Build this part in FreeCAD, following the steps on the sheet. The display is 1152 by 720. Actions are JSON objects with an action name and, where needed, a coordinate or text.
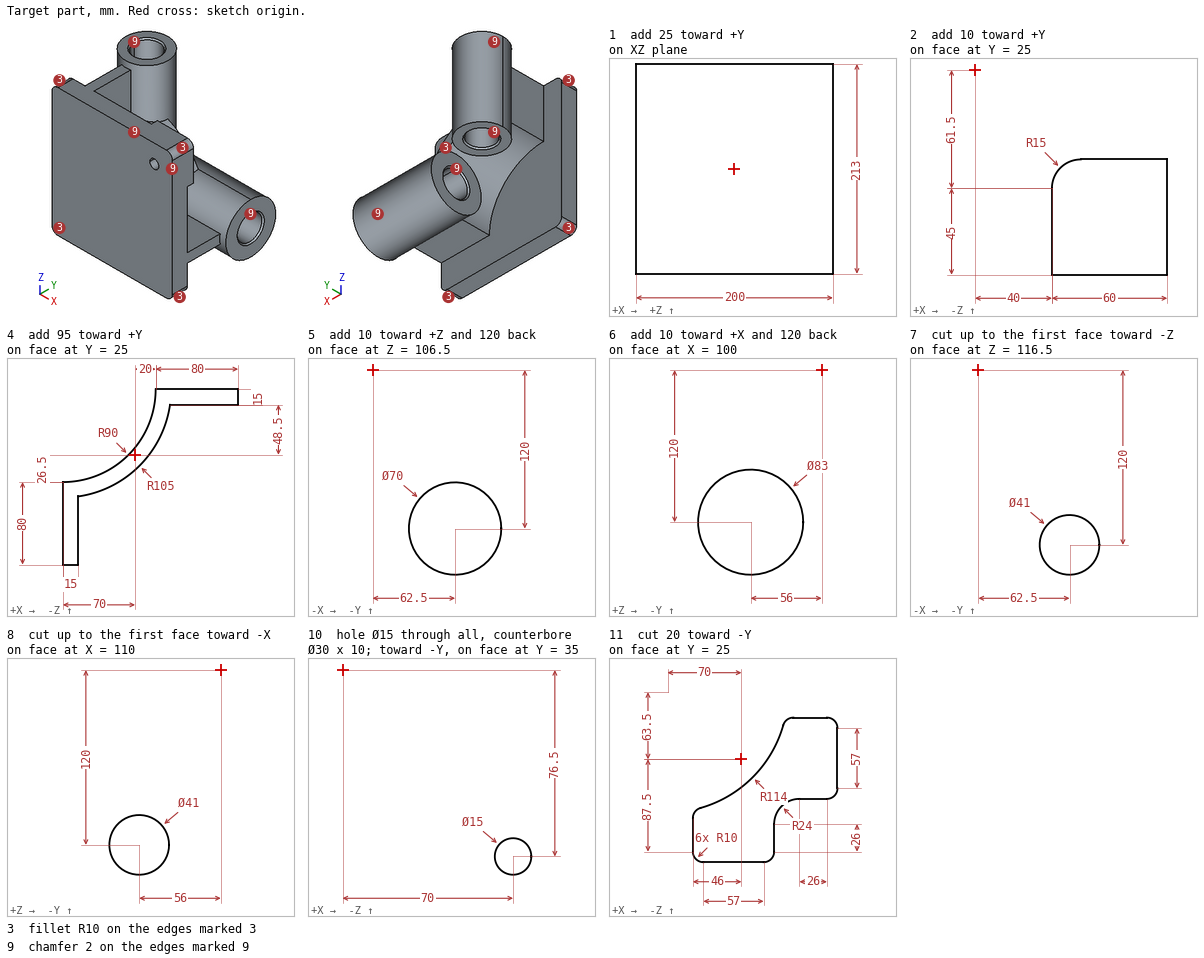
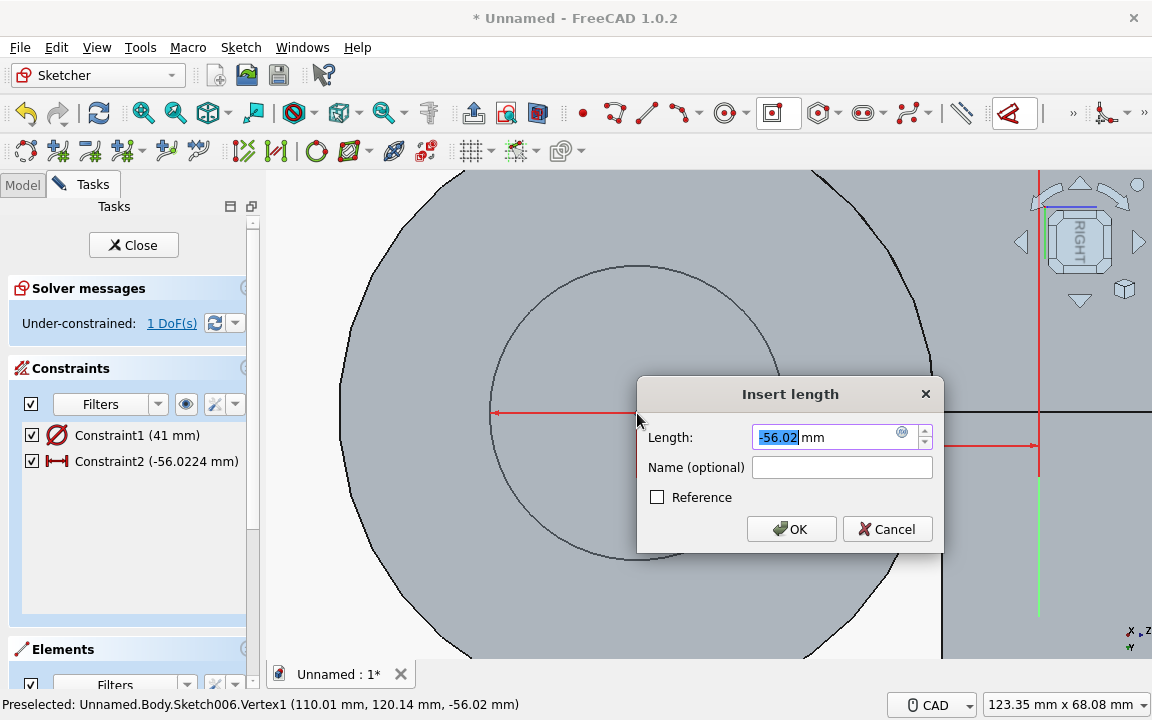
{"action": "type", "text": "-56"}
{"action": "key", "text": "Return"}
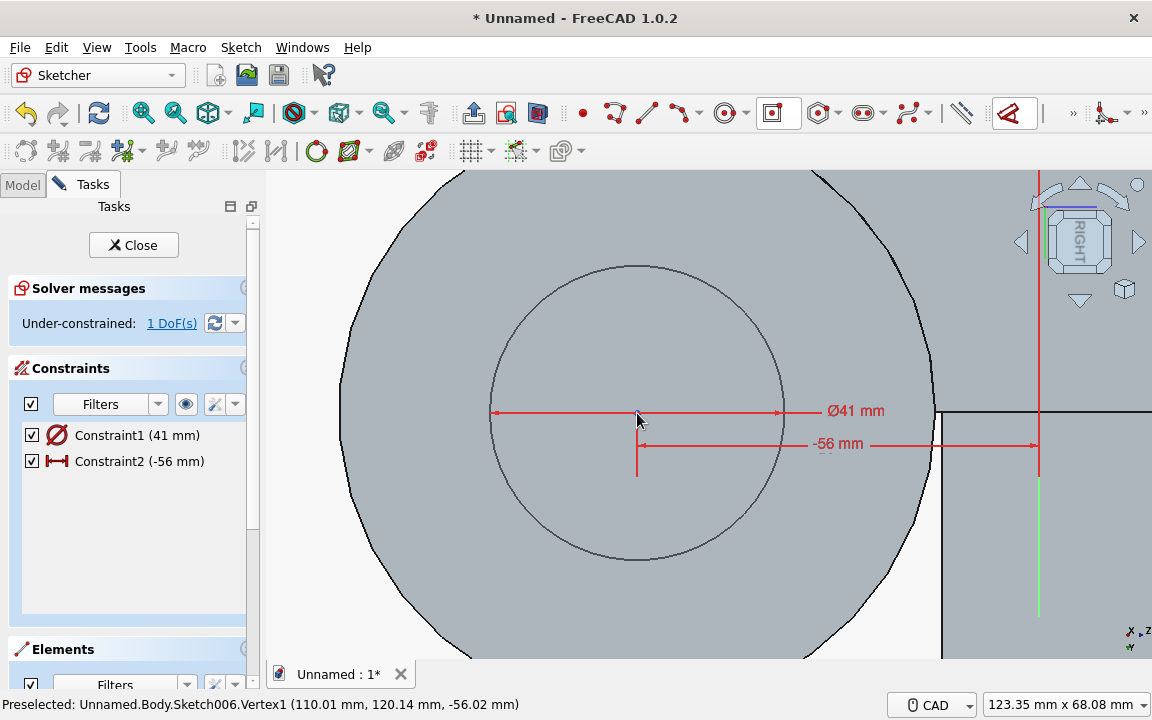
{"action": "left_click", "coordinate": [637, 413]}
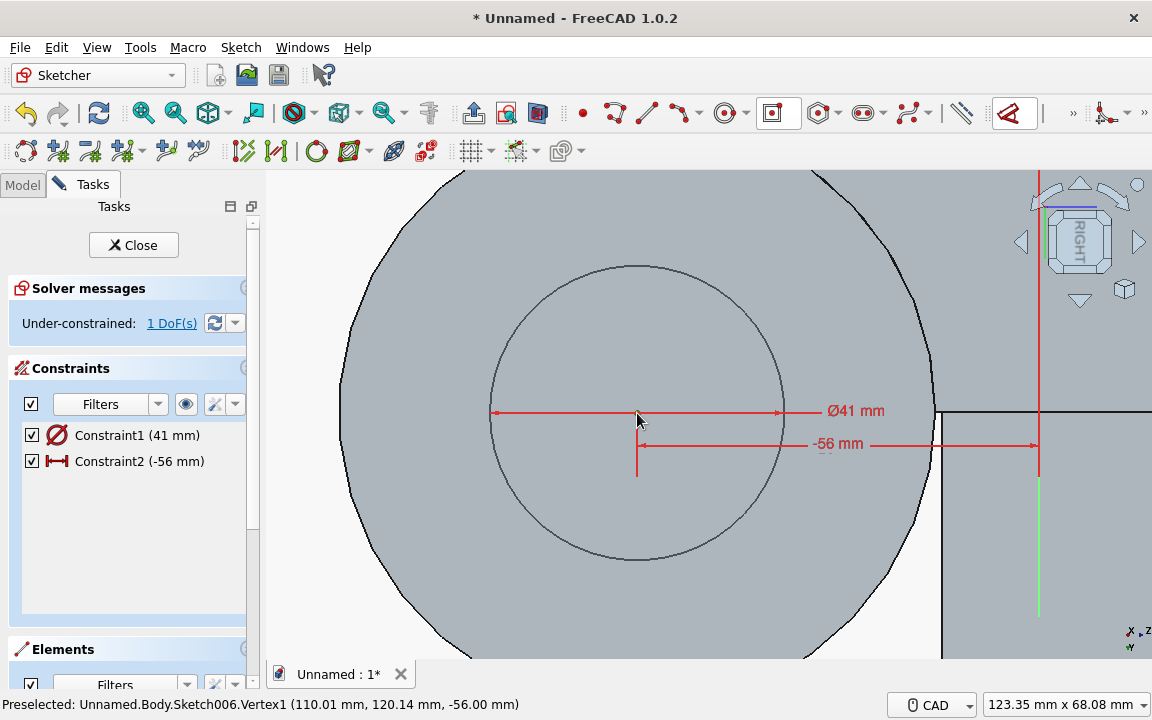
{"action": "left_click", "coordinate": [1032, 114]}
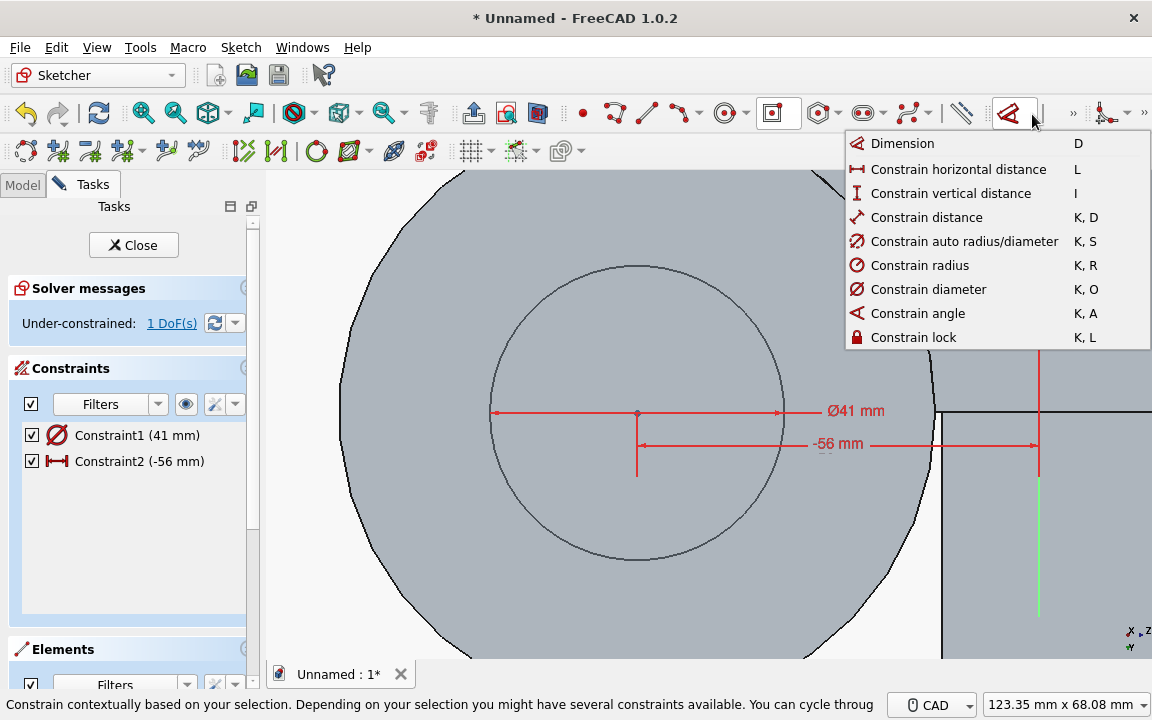
{"action": "left_click", "coordinate": [998, 193]}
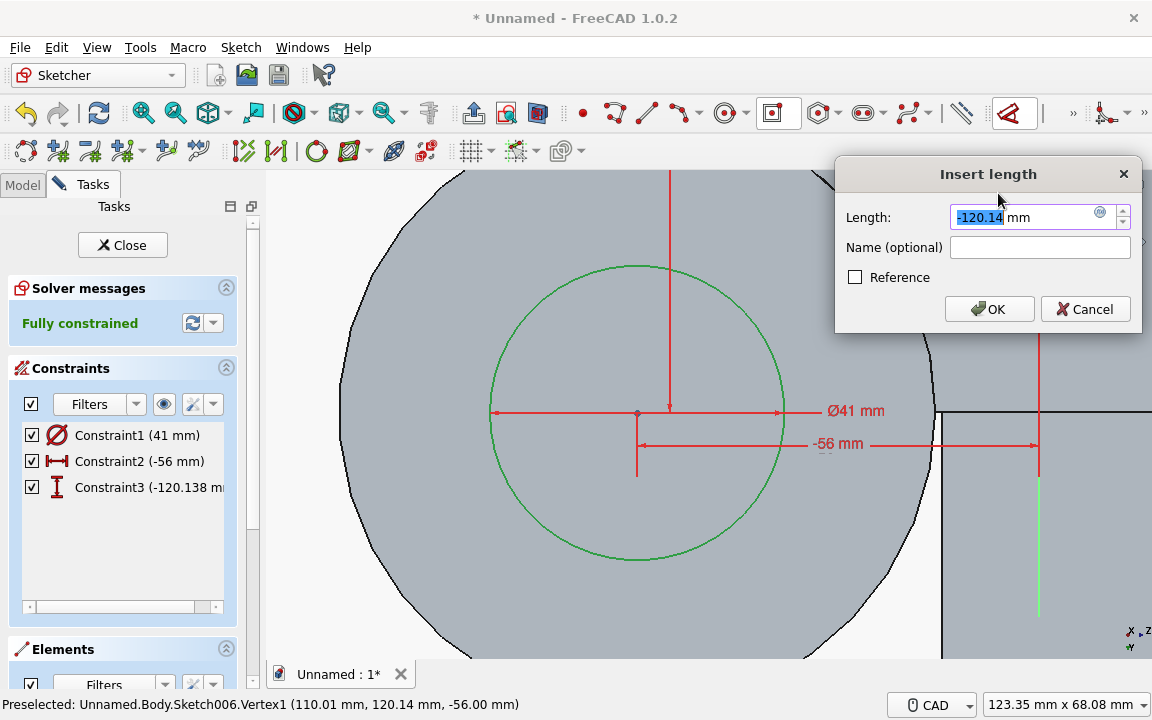
{"action": "type", "text": "-120"}
{"action": "key", "text": "Return"}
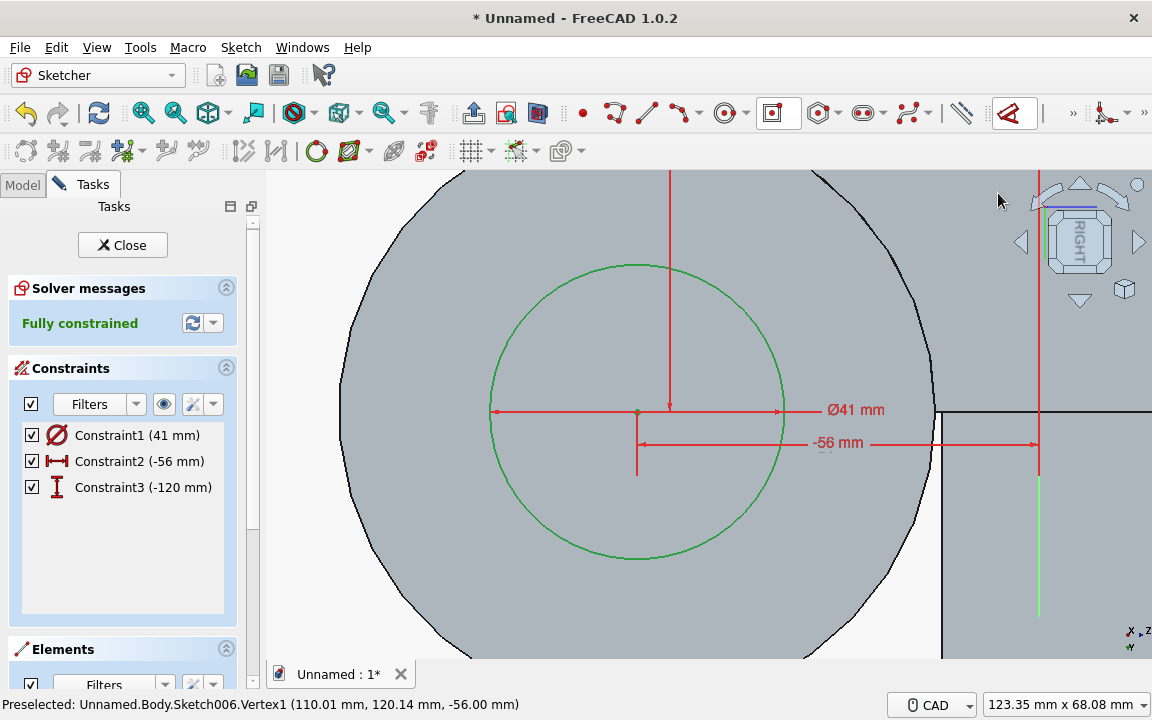
{"action": "left_click", "coordinate": [123, 245]}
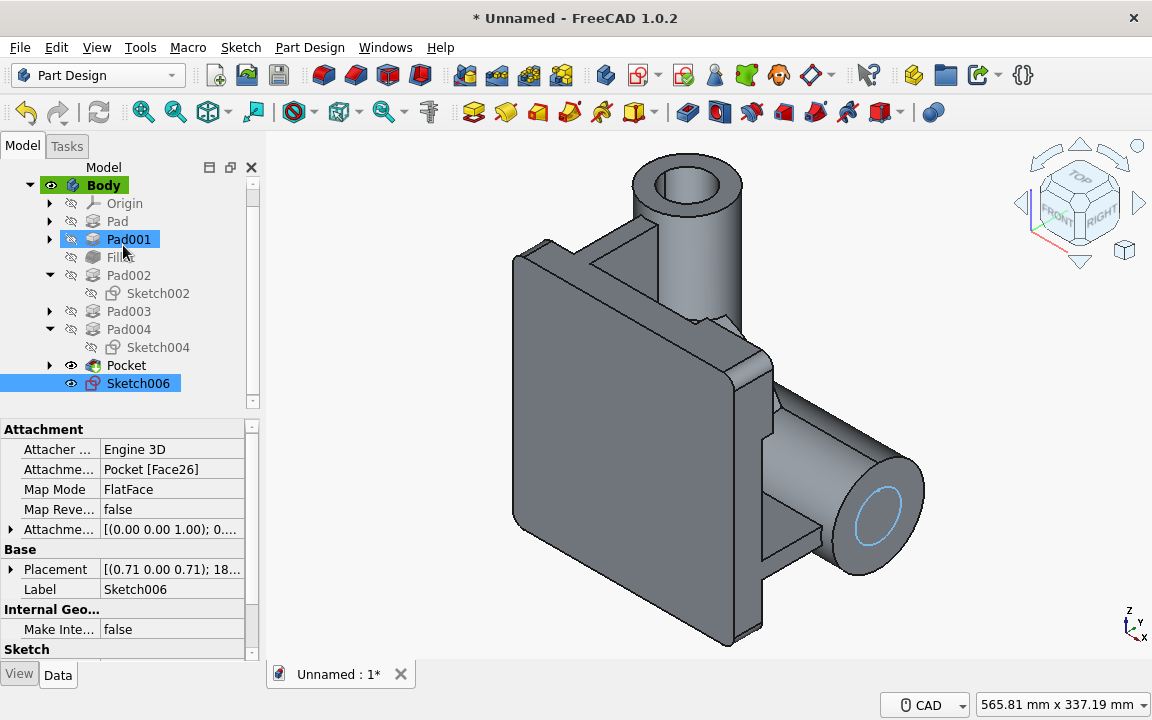
{"action": "left_click", "coordinate": [688, 112]}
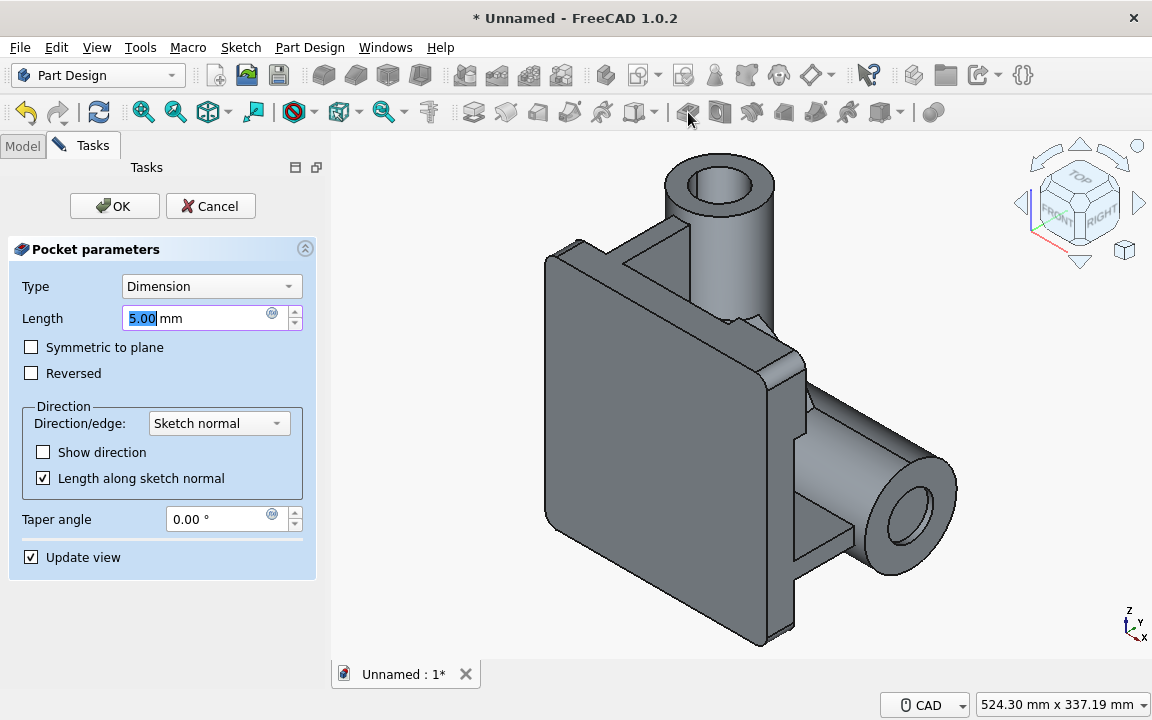
{"action": "left_click", "coordinate": [212, 286]}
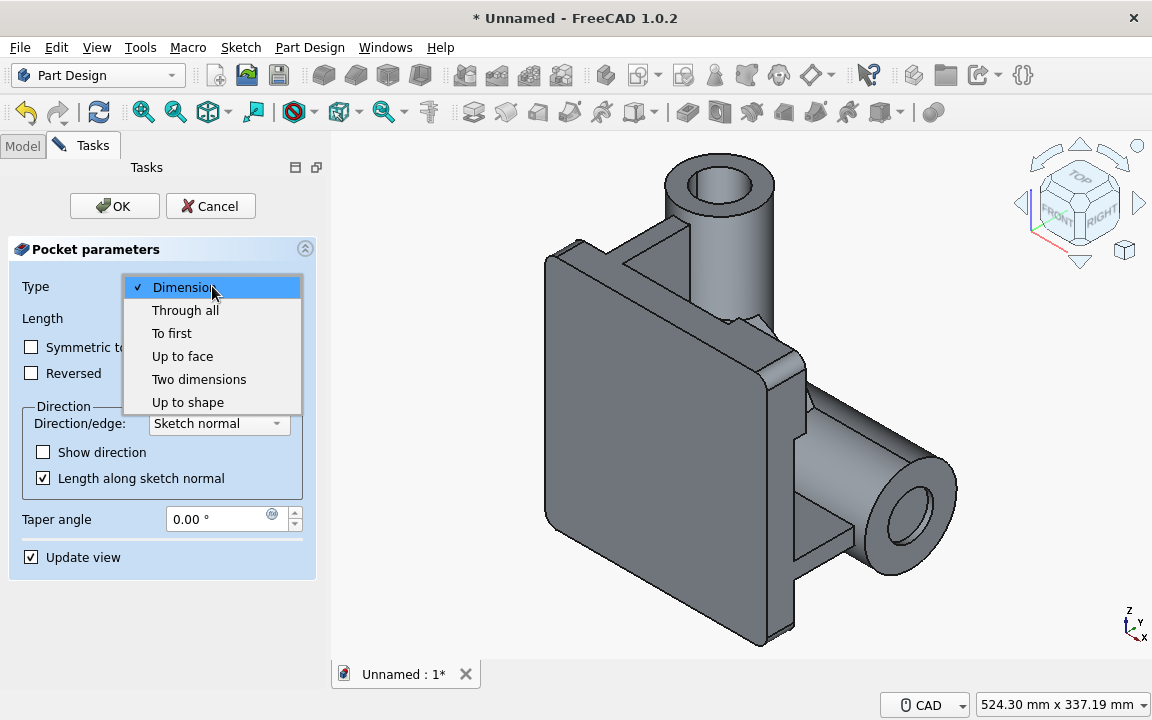
{"action": "left_click", "coordinate": [212, 334]}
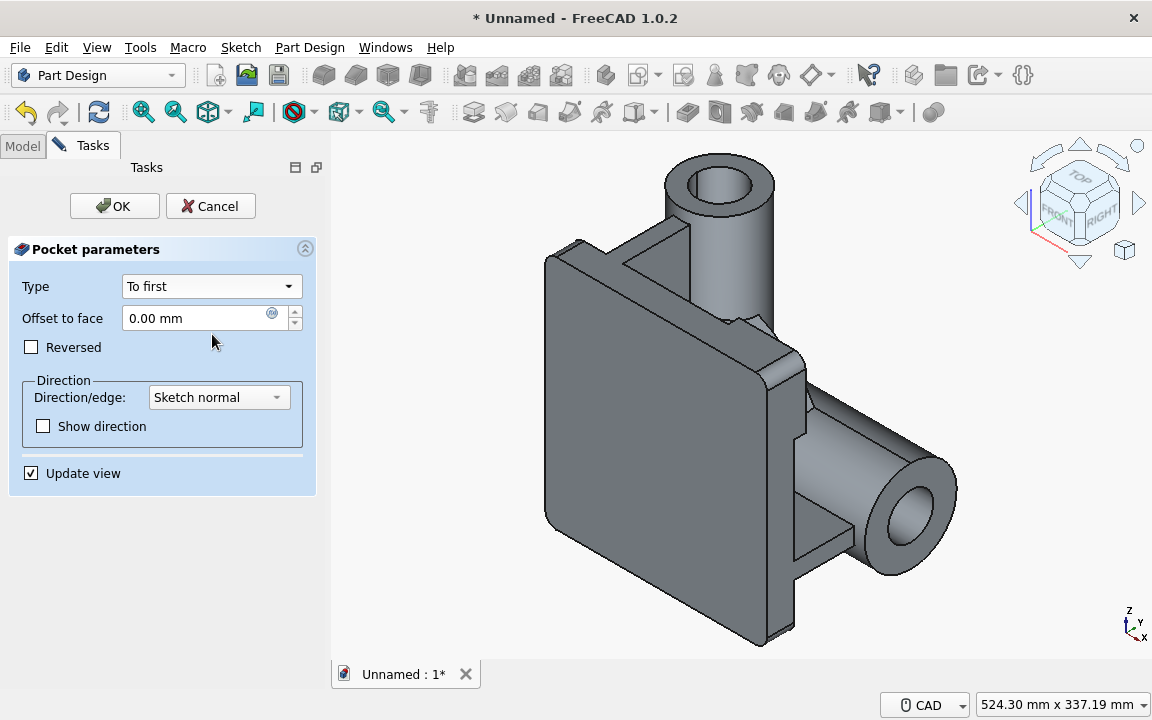
{"action": "left_click", "coordinate": [115, 206]}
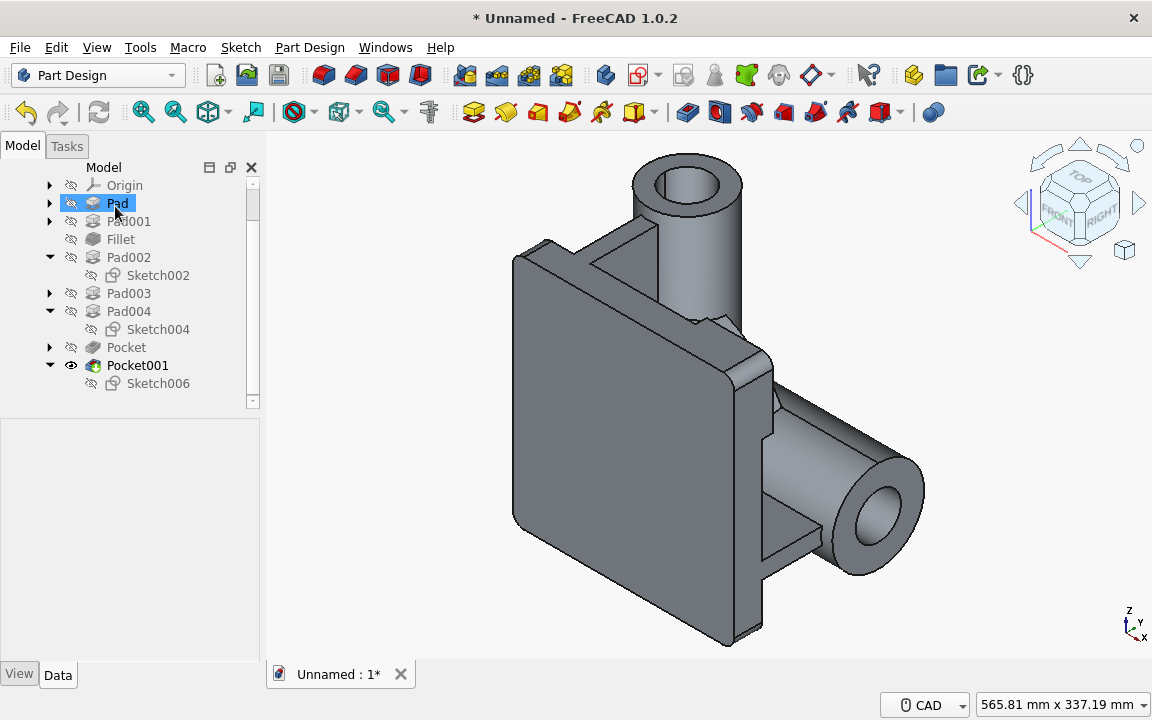
{"action": "left_click", "coordinate": [716, 176]}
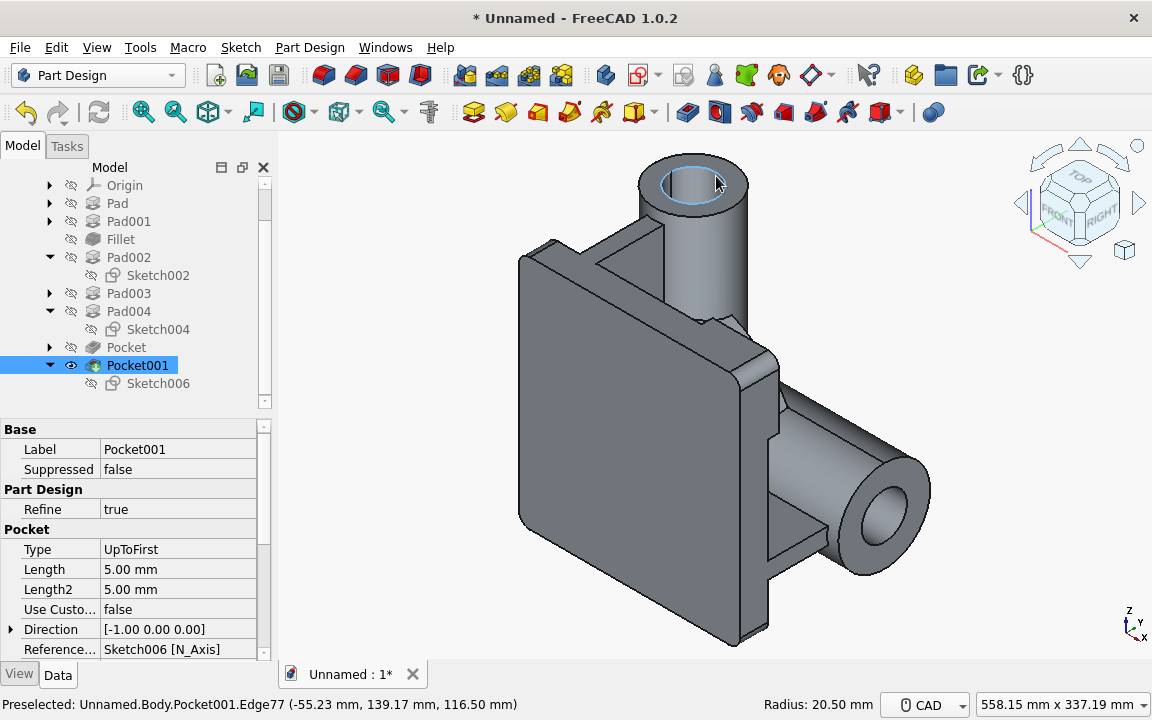
{"action": "left_click", "coordinate": [884, 541], "text": "ctrl"}